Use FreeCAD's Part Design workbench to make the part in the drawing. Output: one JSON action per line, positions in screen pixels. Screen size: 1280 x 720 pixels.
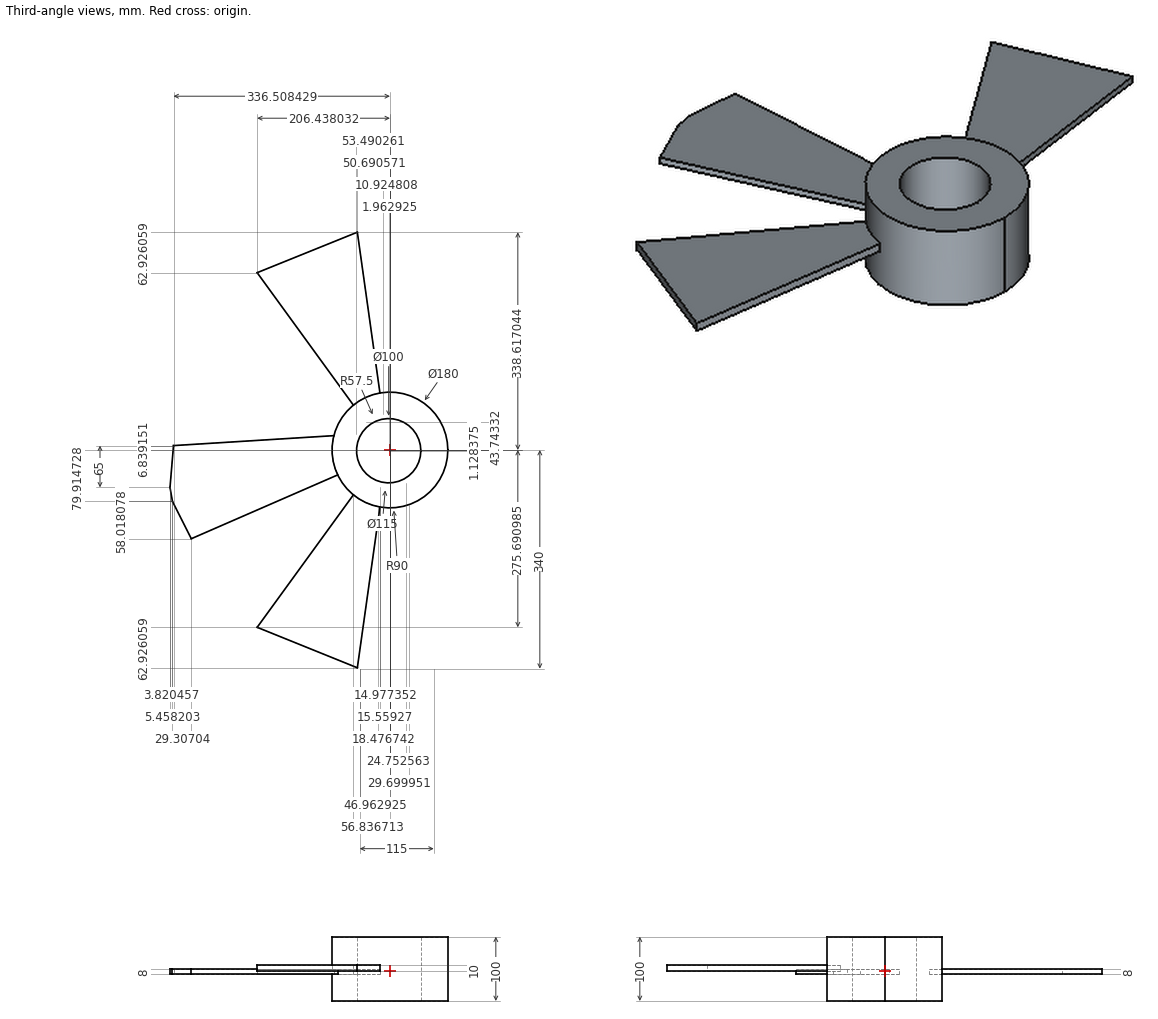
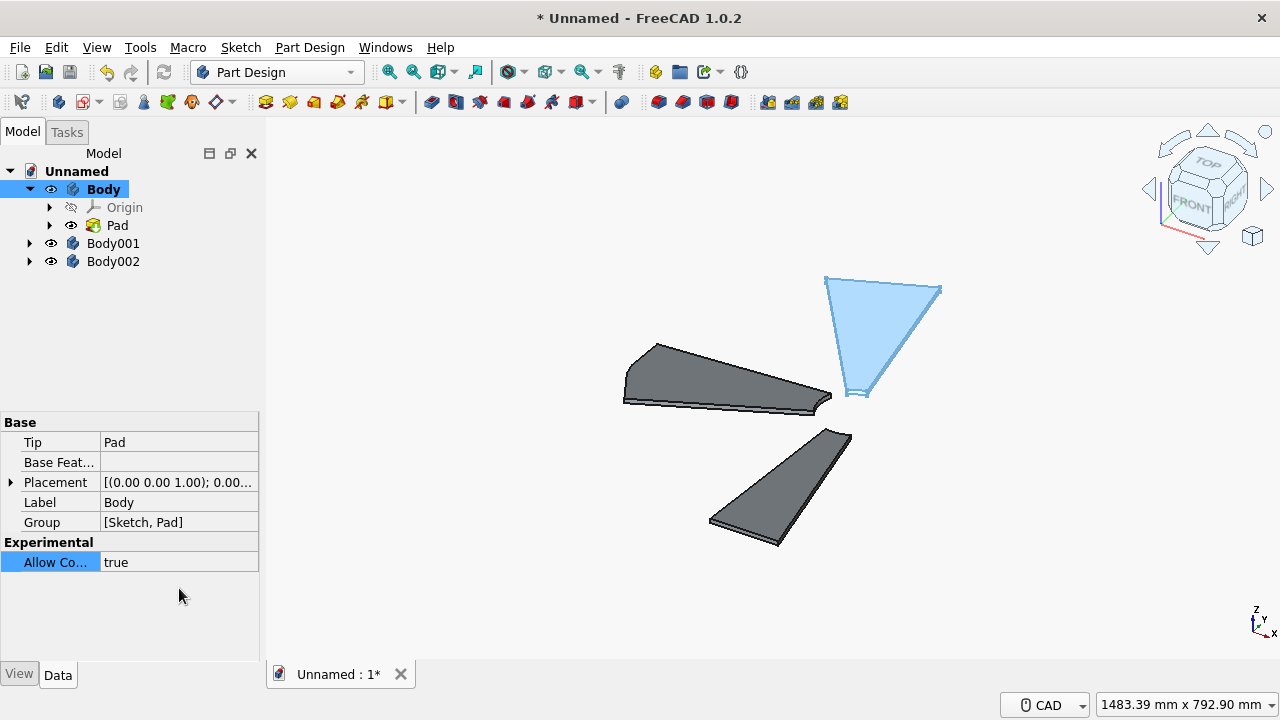
{"action": "left_click", "coordinate": [96, 243]}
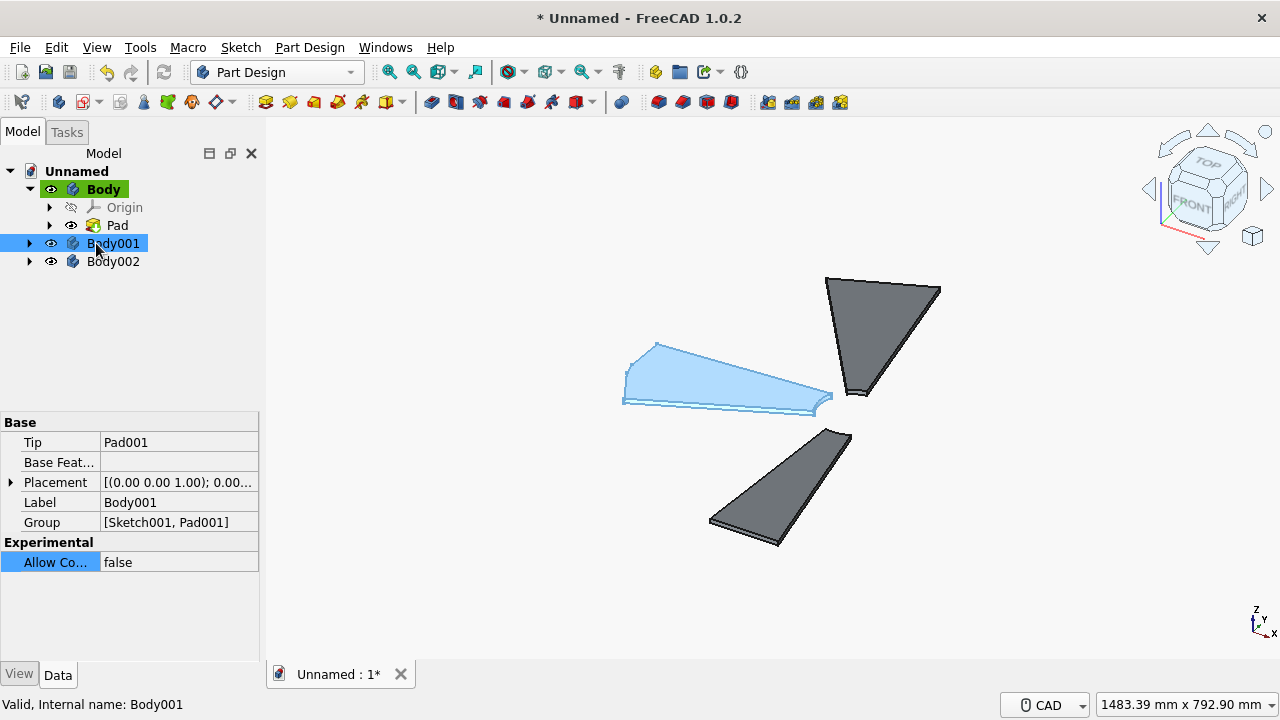
{"action": "left_click", "coordinate": [622, 102]}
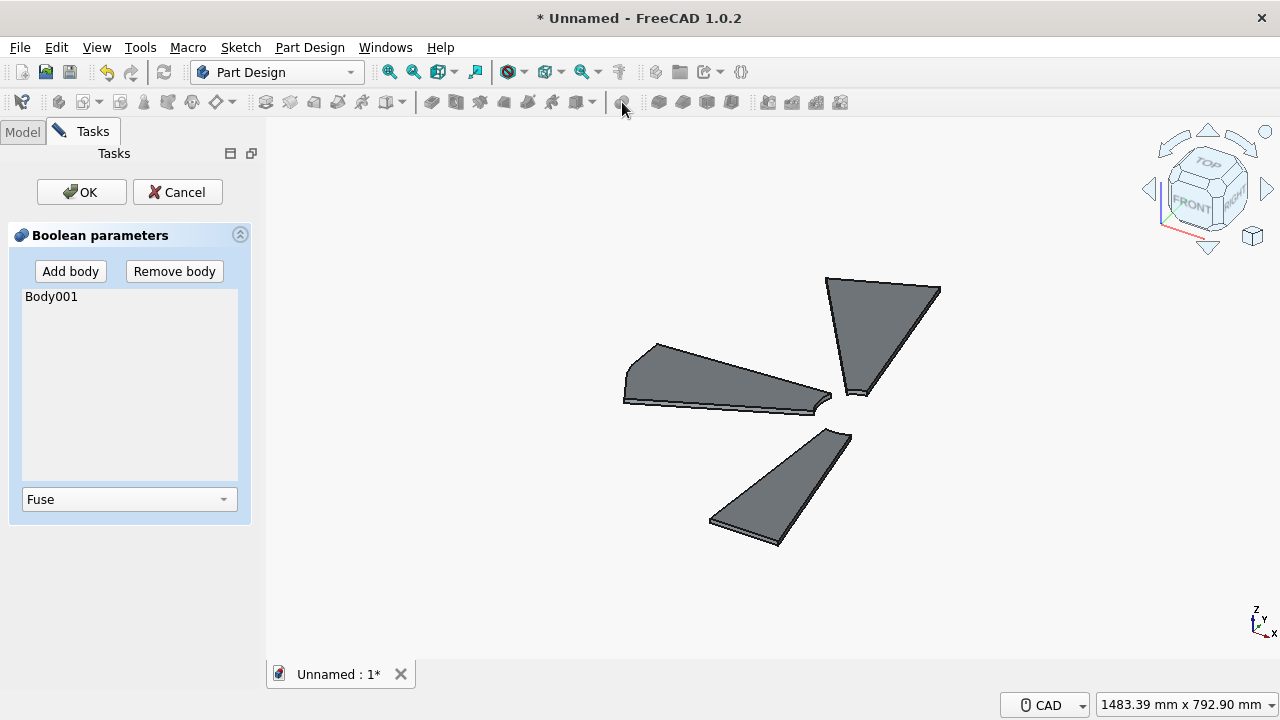
{"action": "left_click", "coordinate": [82, 192]}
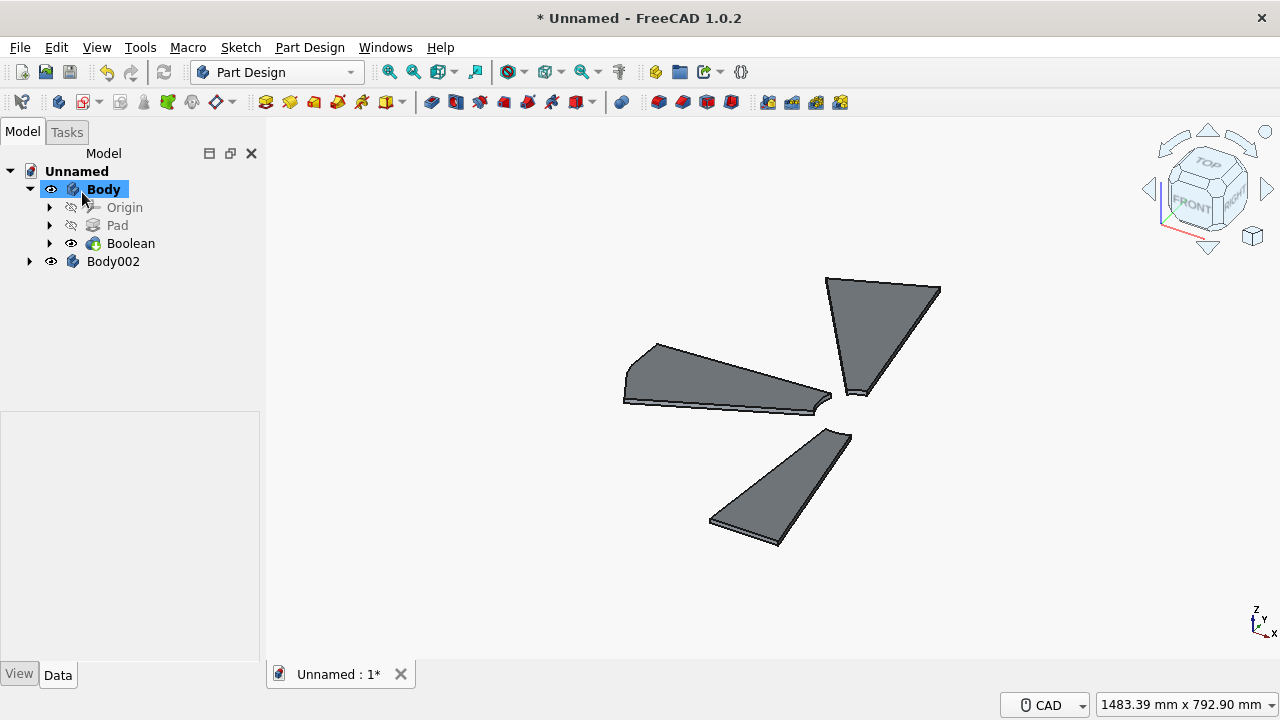
{"action": "left_click", "coordinate": [390, 72]}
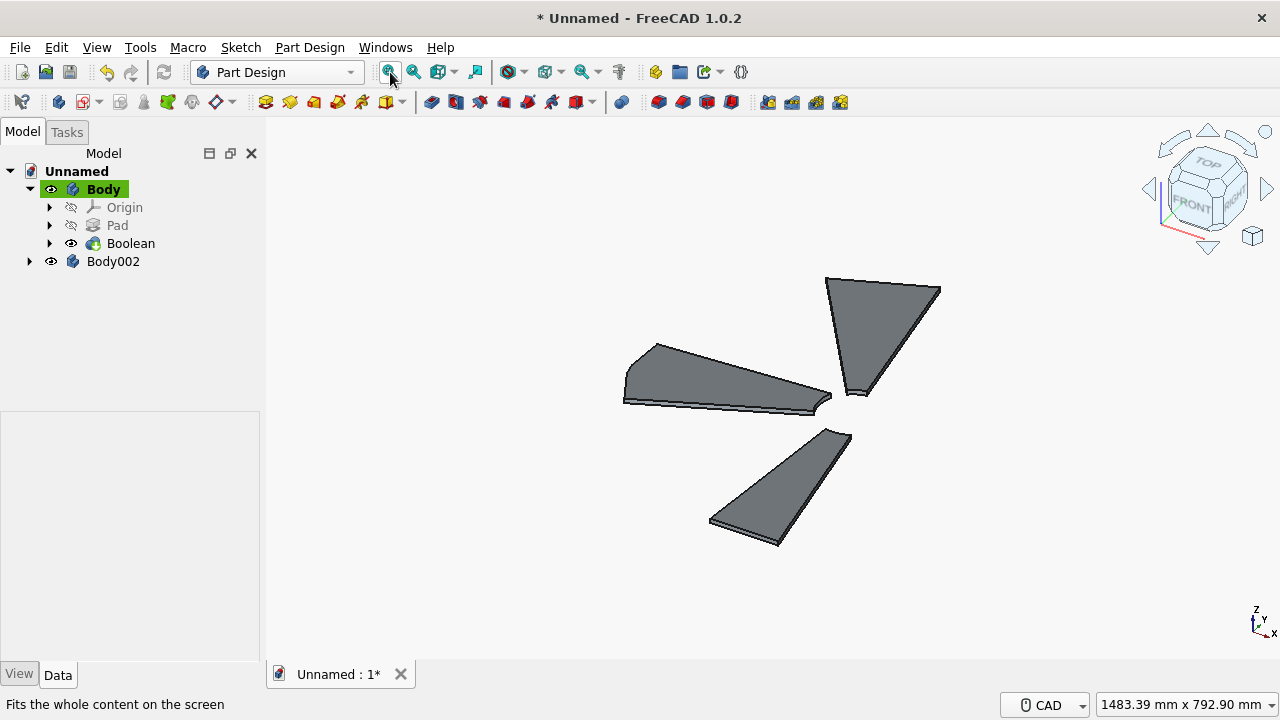
{"action": "left_click", "coordinate": [96, 261]}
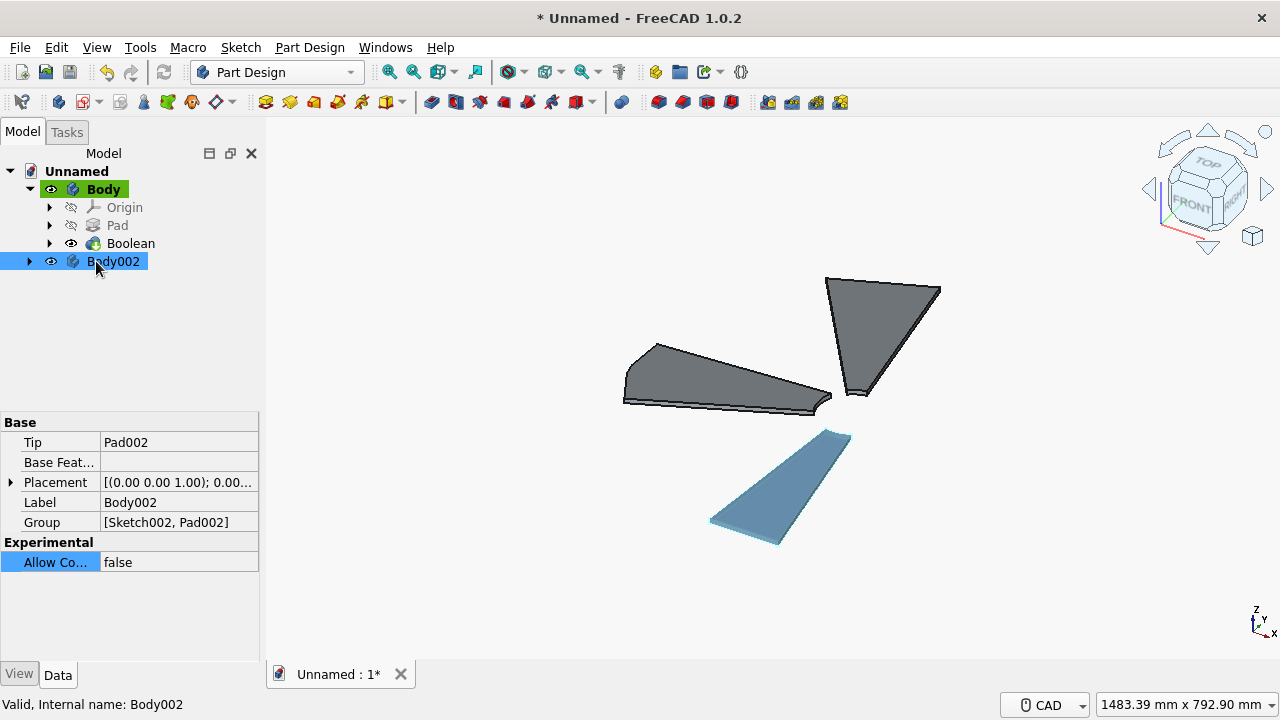
{"action": "left_click", "coordinate": [622, 102]}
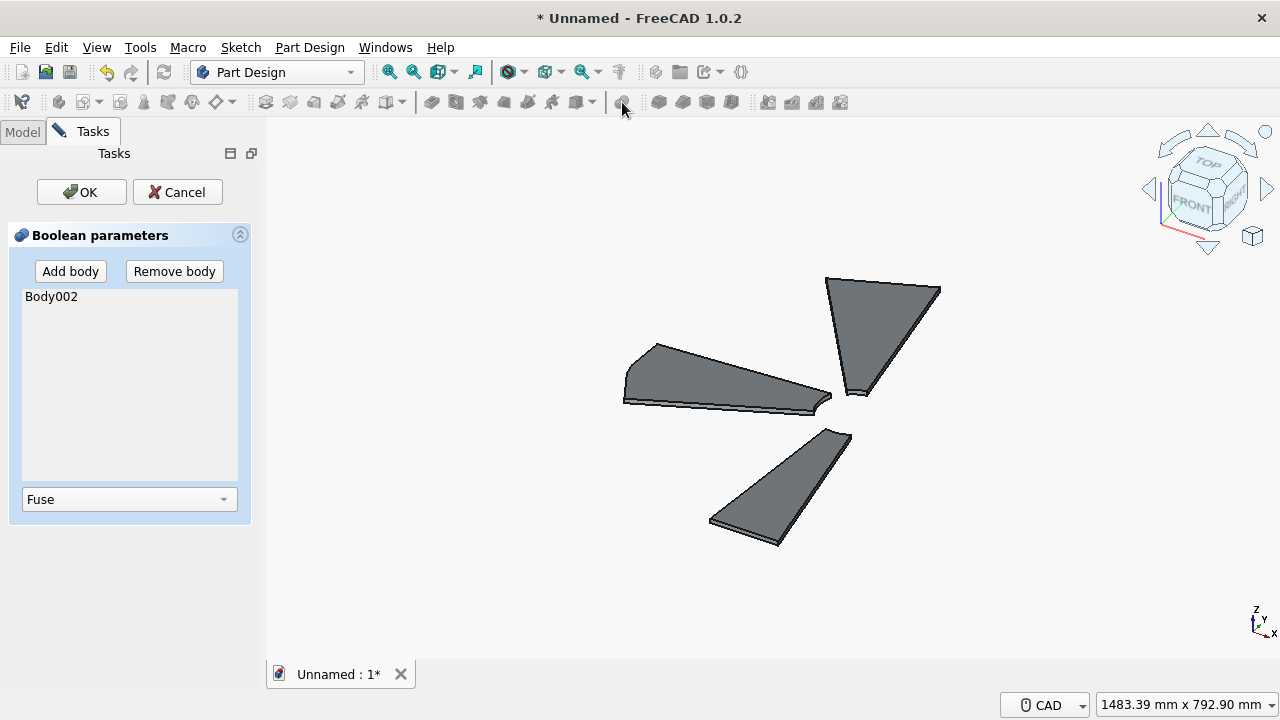
{"action": "left_click", "coordinate": [82, 192]}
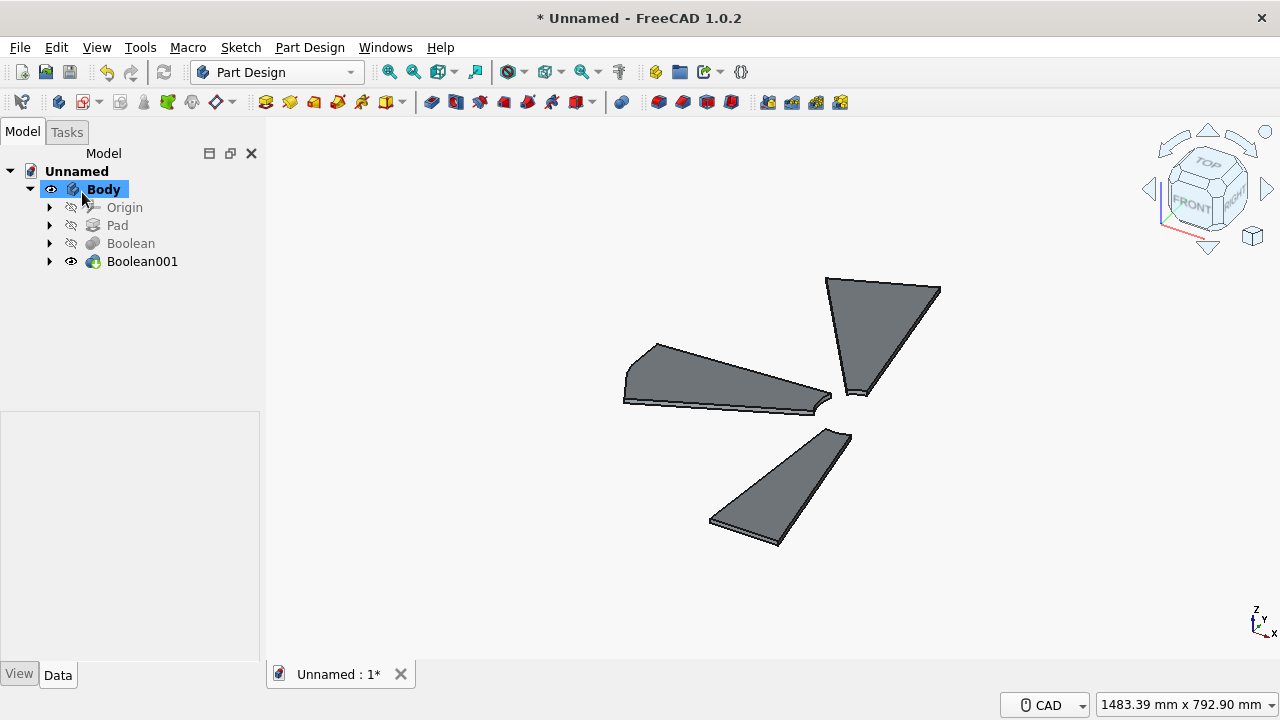
{"action": "left_click", "coordinate": [669, 376]}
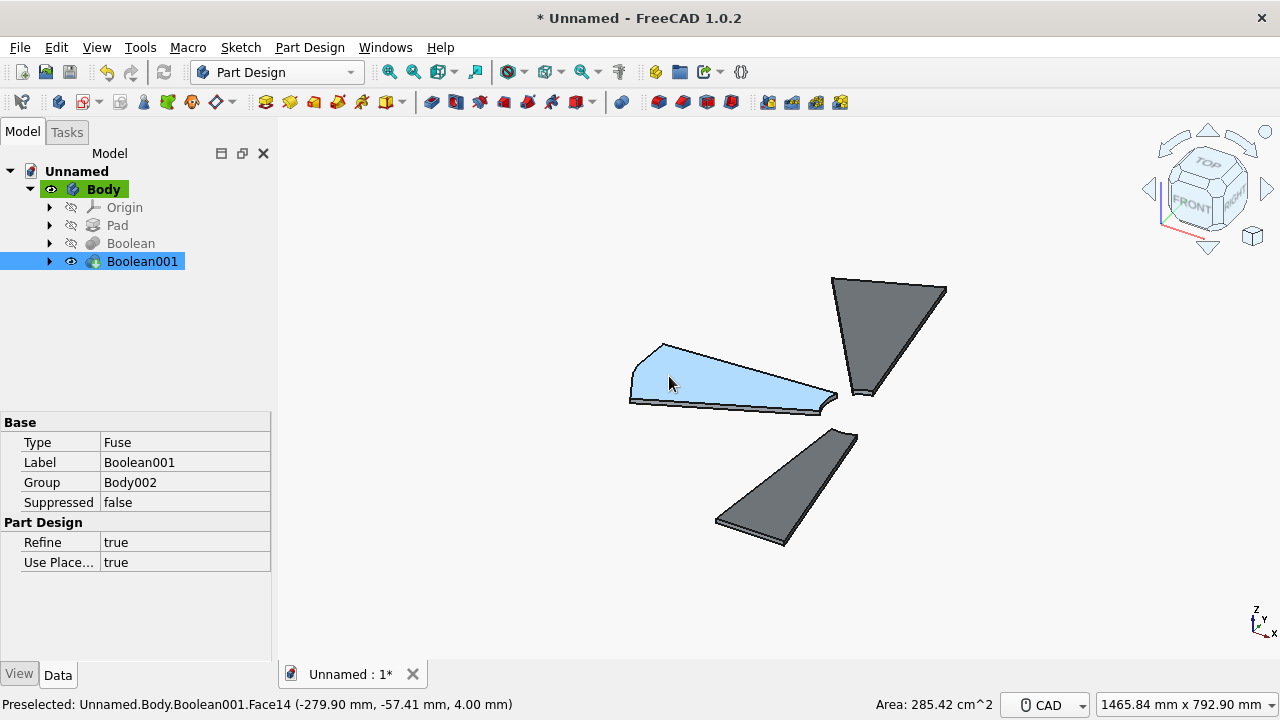
{"action": "left_click", "coordinate": [84, 102]}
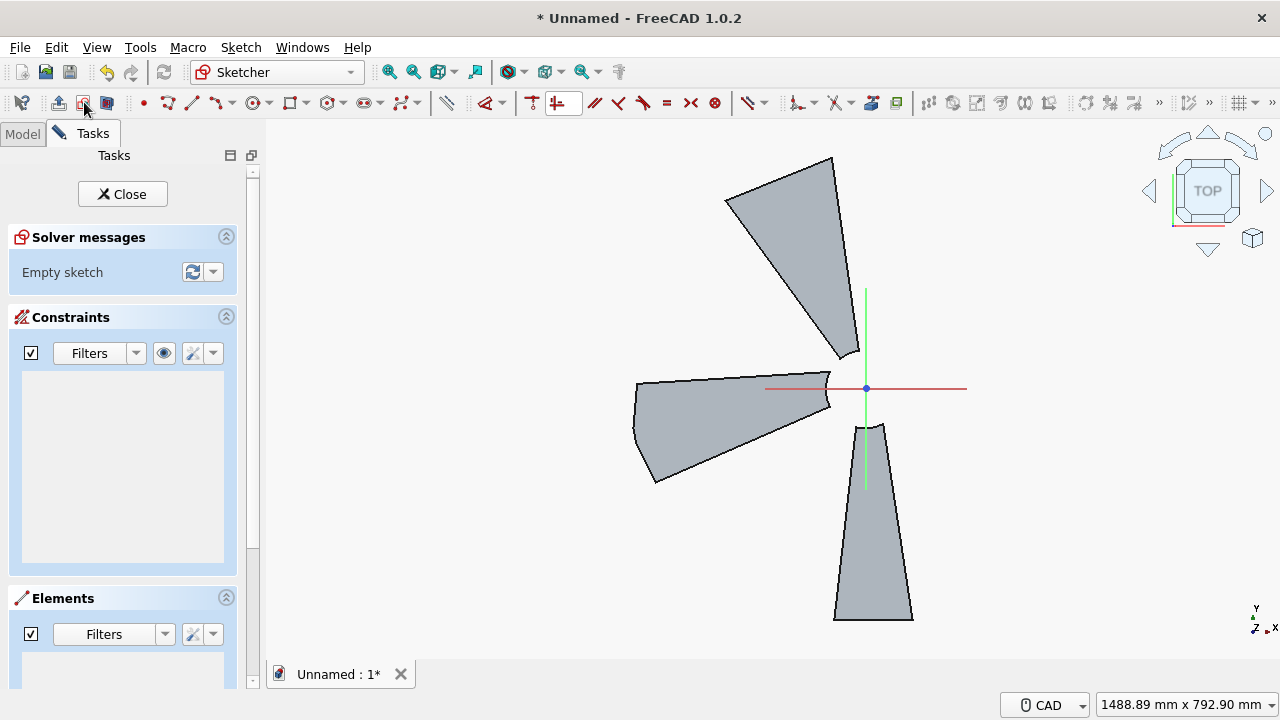
{"action": "scroll", "coordinate": [960, 388], "scroll_direction": "up", "scroll_amount": 5}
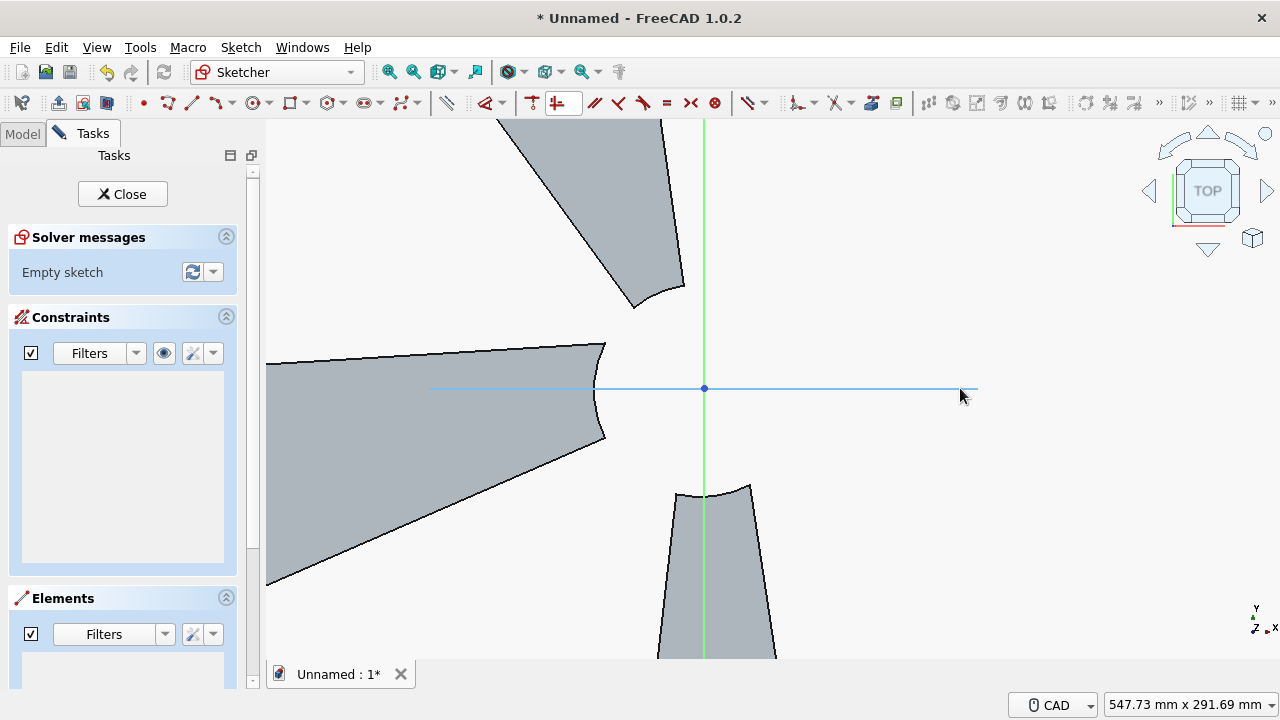
{"action": "left_click", "coordinate": [254, 104]}